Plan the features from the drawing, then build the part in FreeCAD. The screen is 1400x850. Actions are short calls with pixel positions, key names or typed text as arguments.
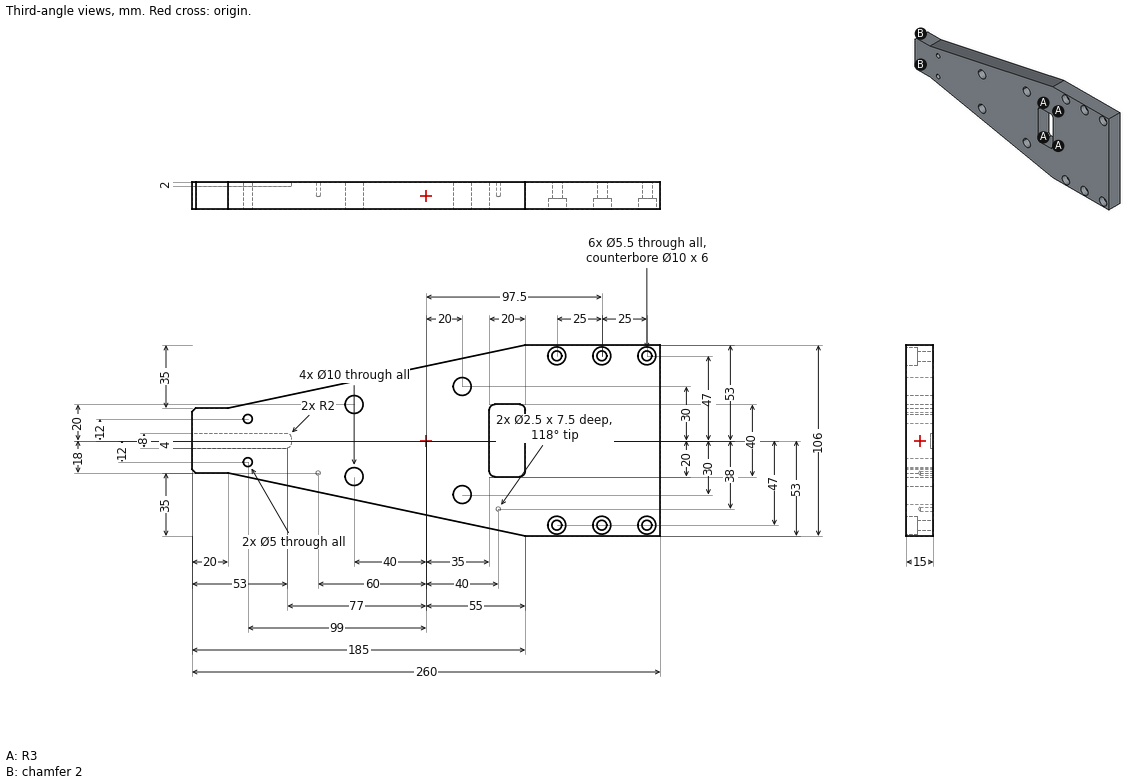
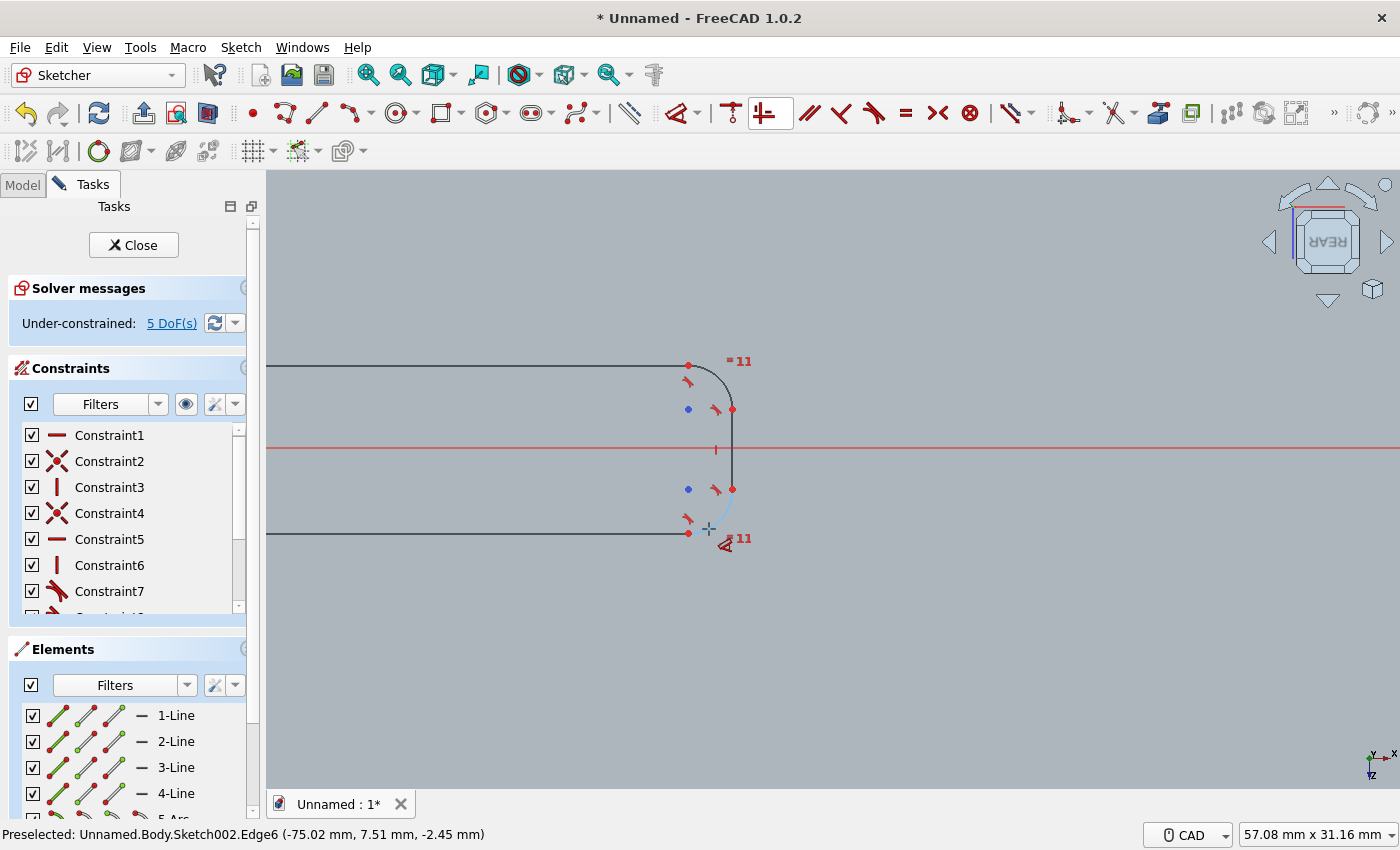
click(708, 529)
click(722, 558)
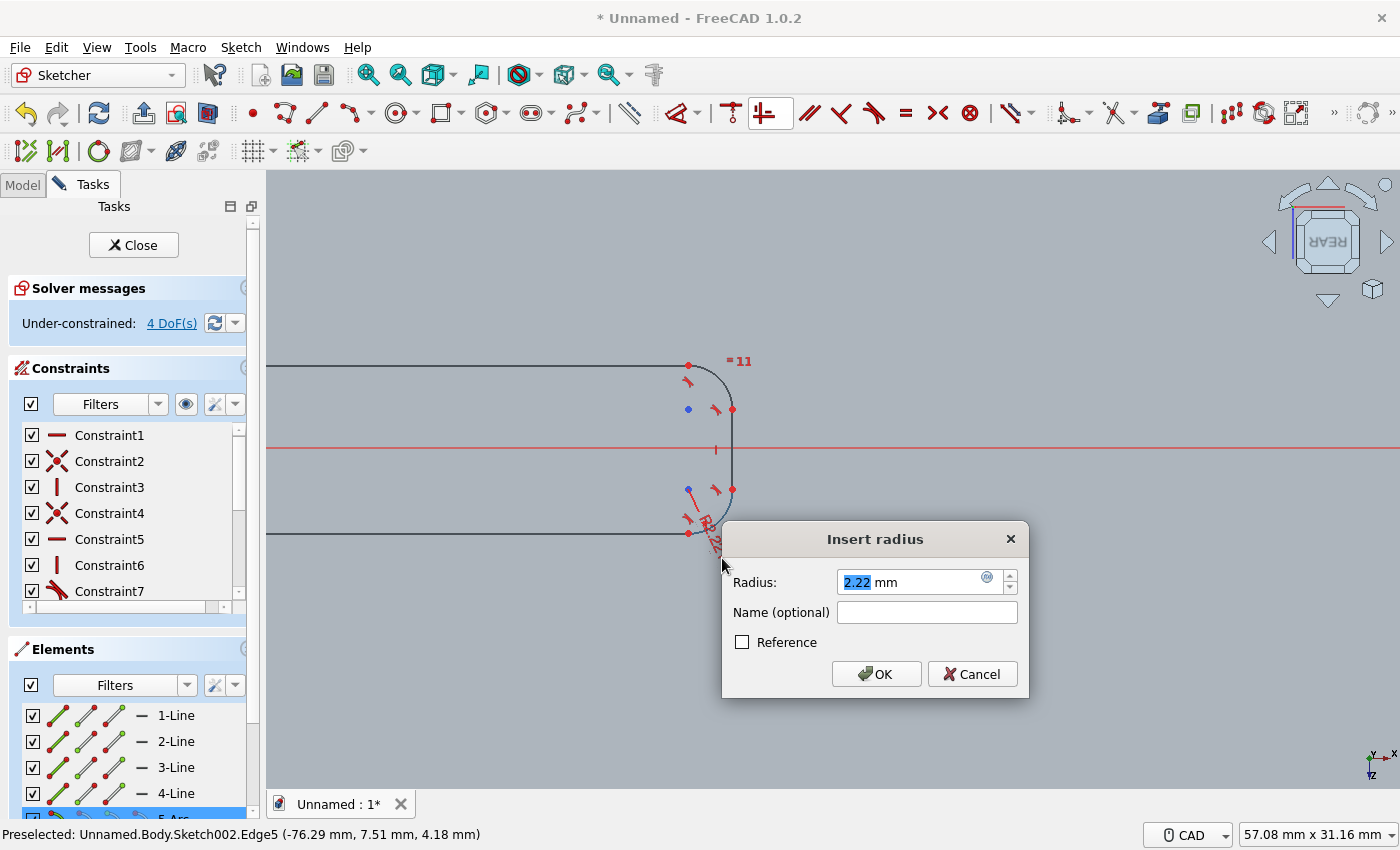
text(2)
key(Return)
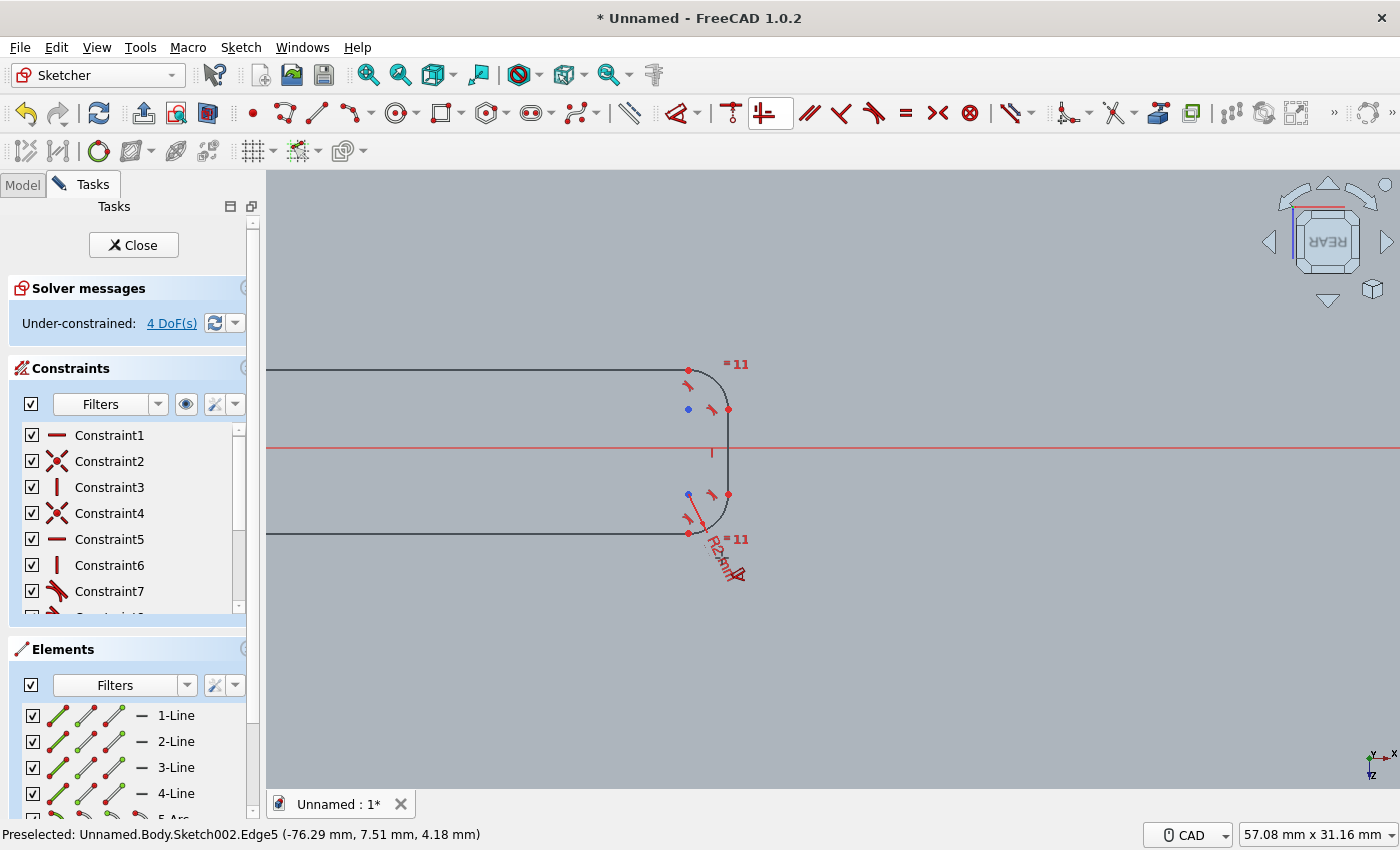
scroll(711, 490, down, 7)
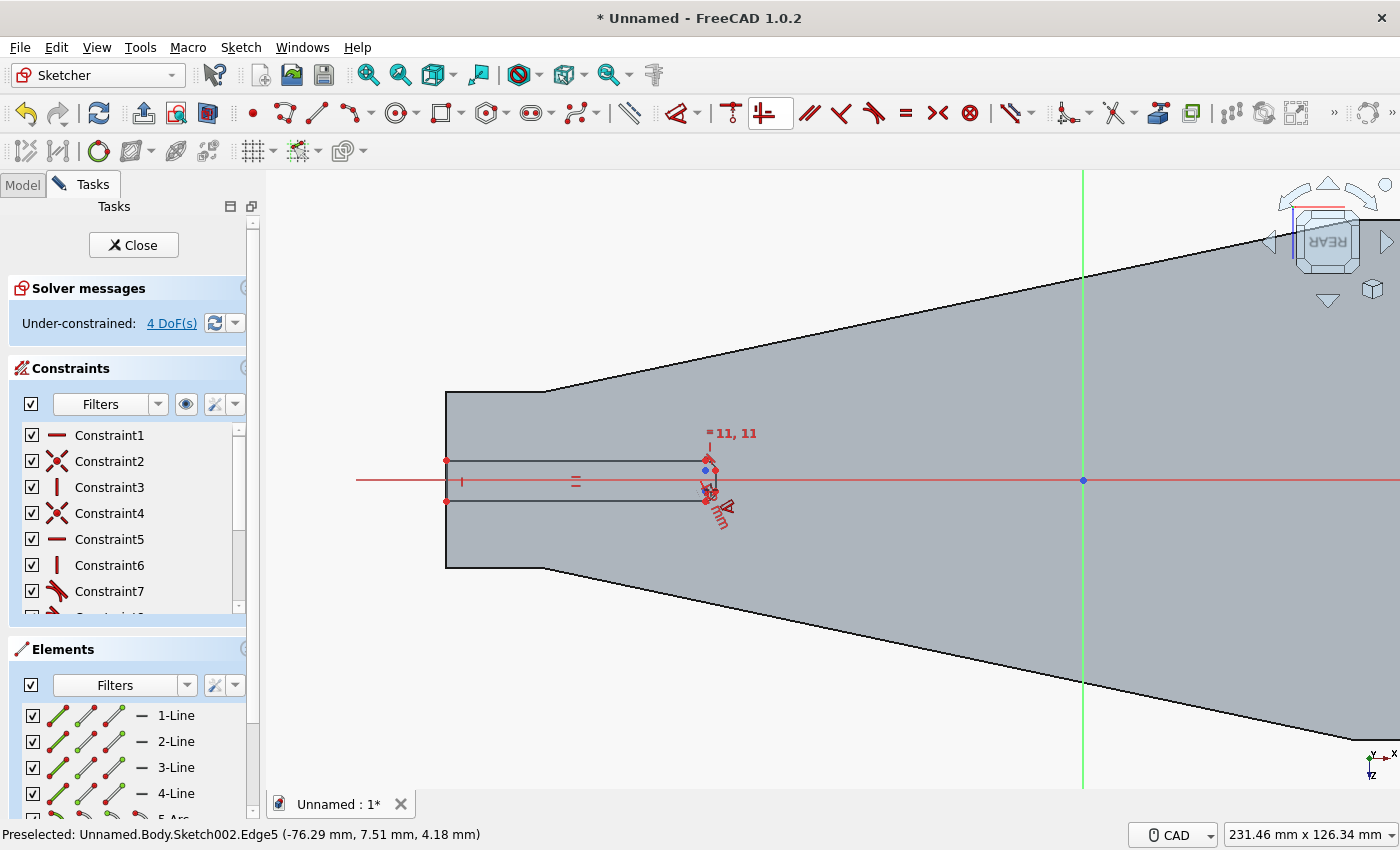
scroll(447, 473, up, 4)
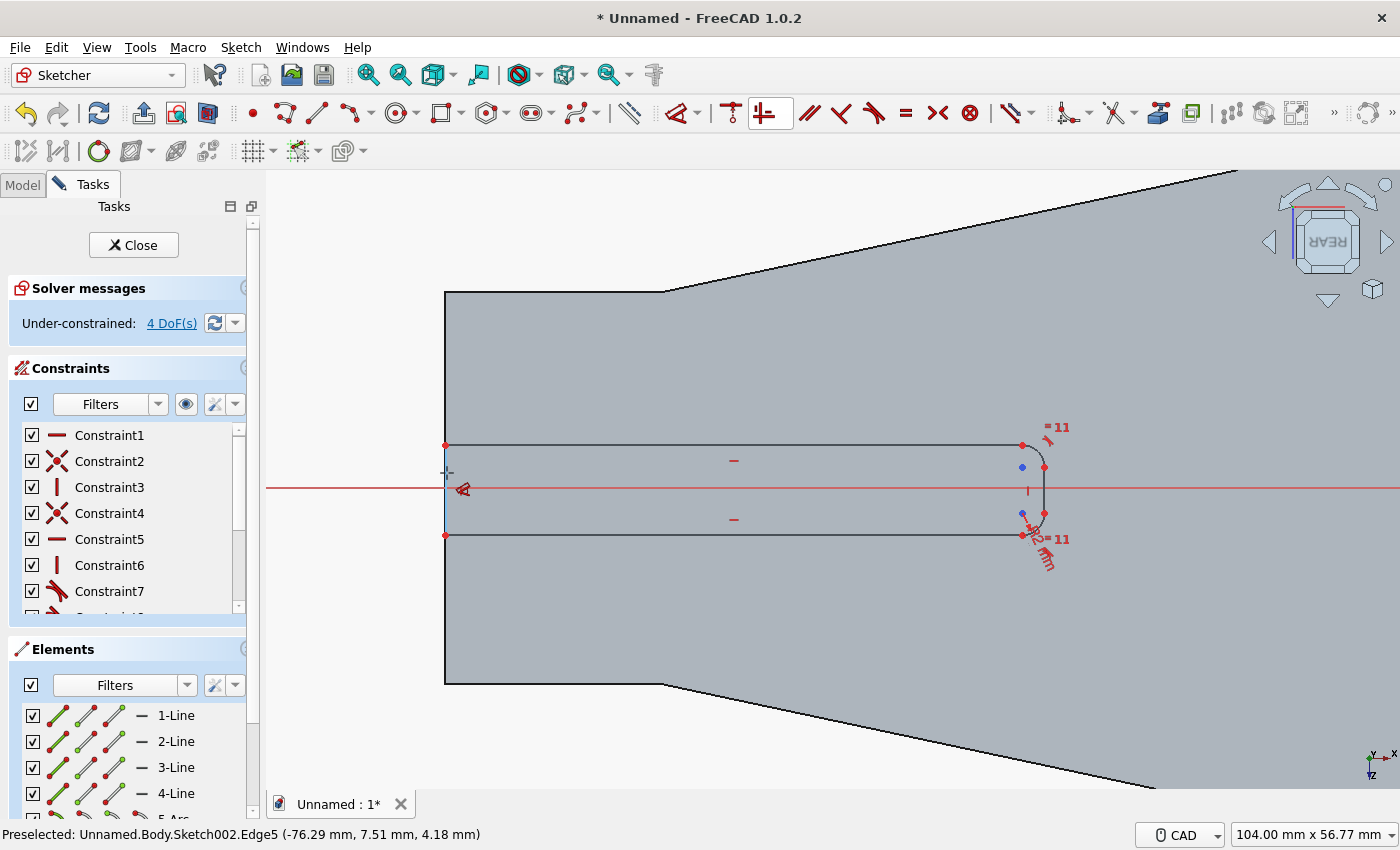
click(446, 472)
click(412, 470)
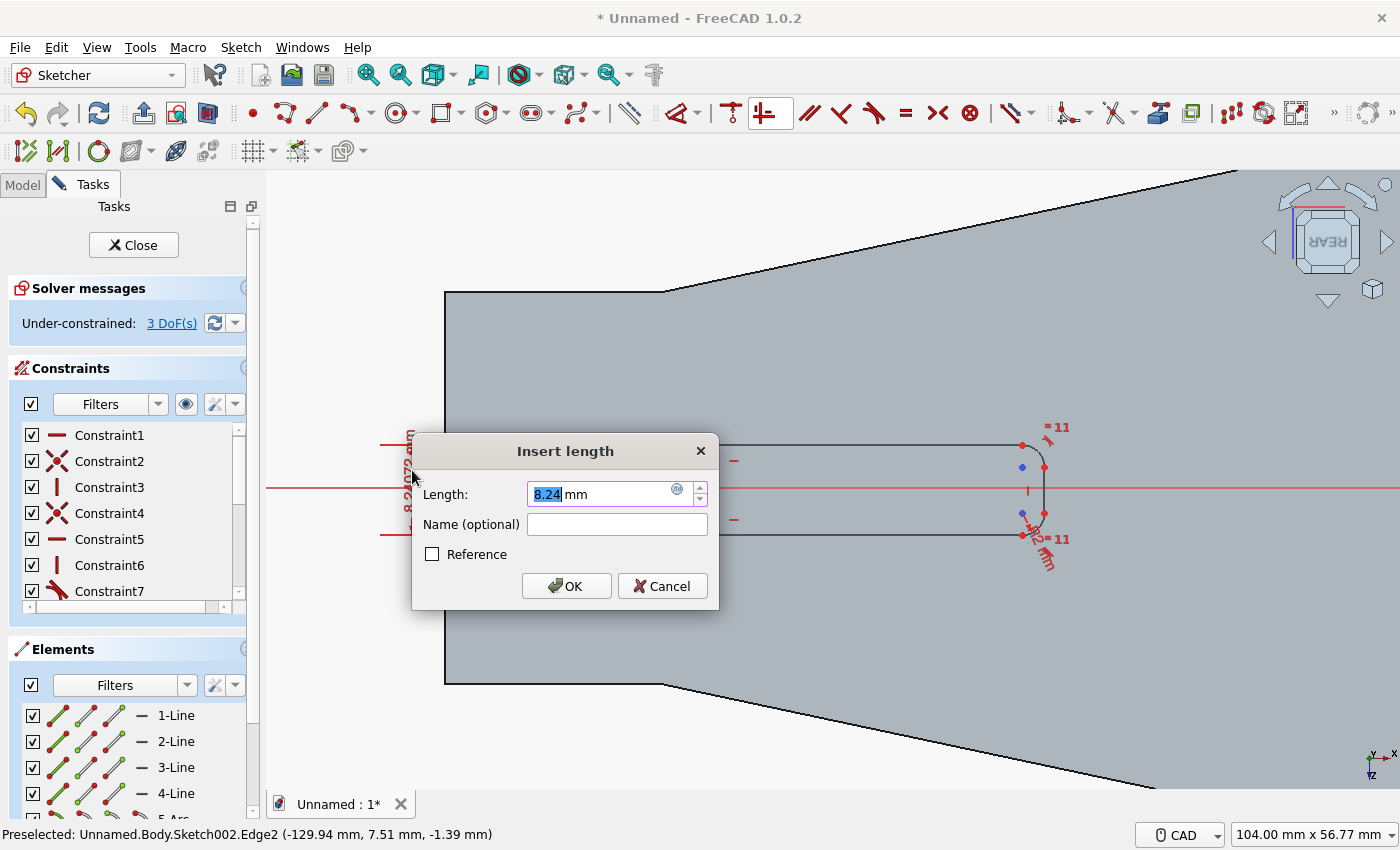
text(8)
key(Return)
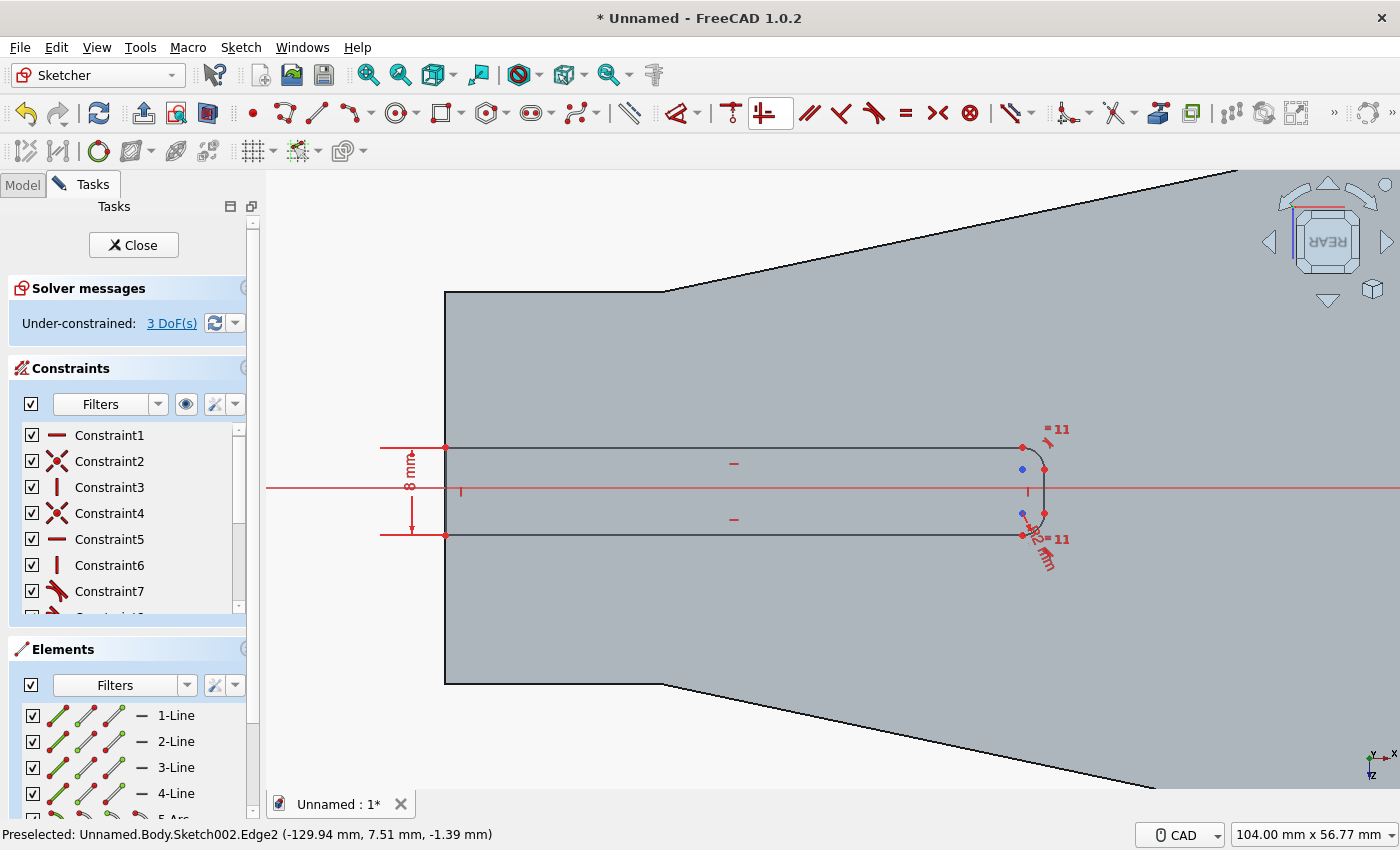
click(850, 448)
click(734, 414)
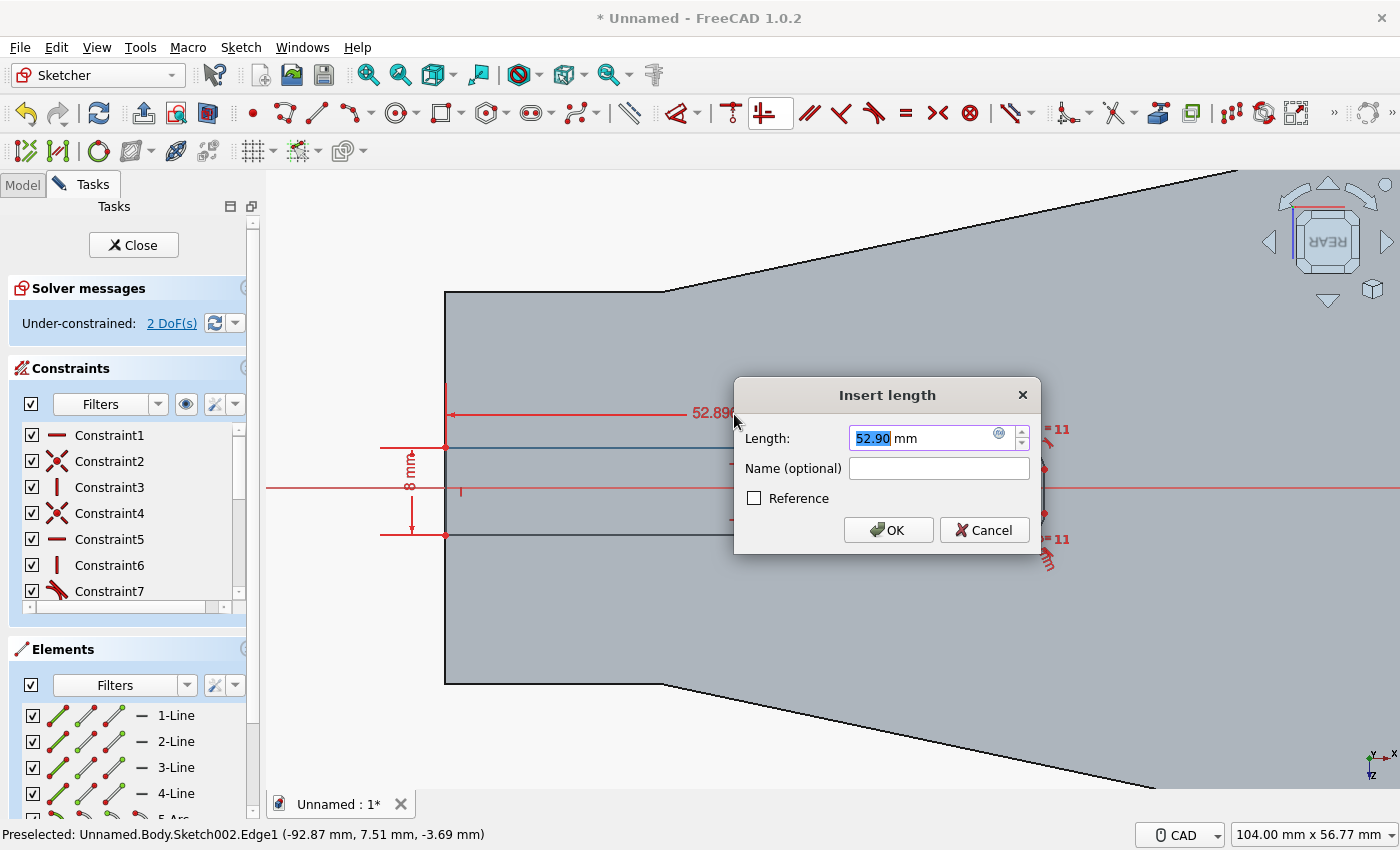
text(53)
key(Return)